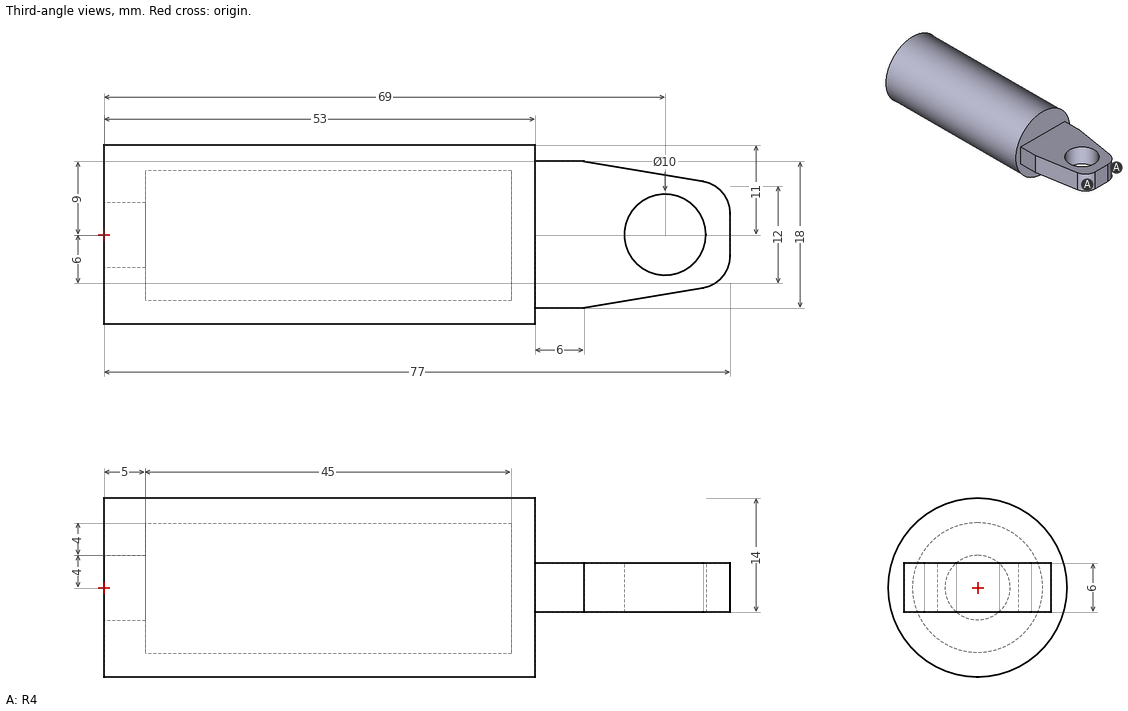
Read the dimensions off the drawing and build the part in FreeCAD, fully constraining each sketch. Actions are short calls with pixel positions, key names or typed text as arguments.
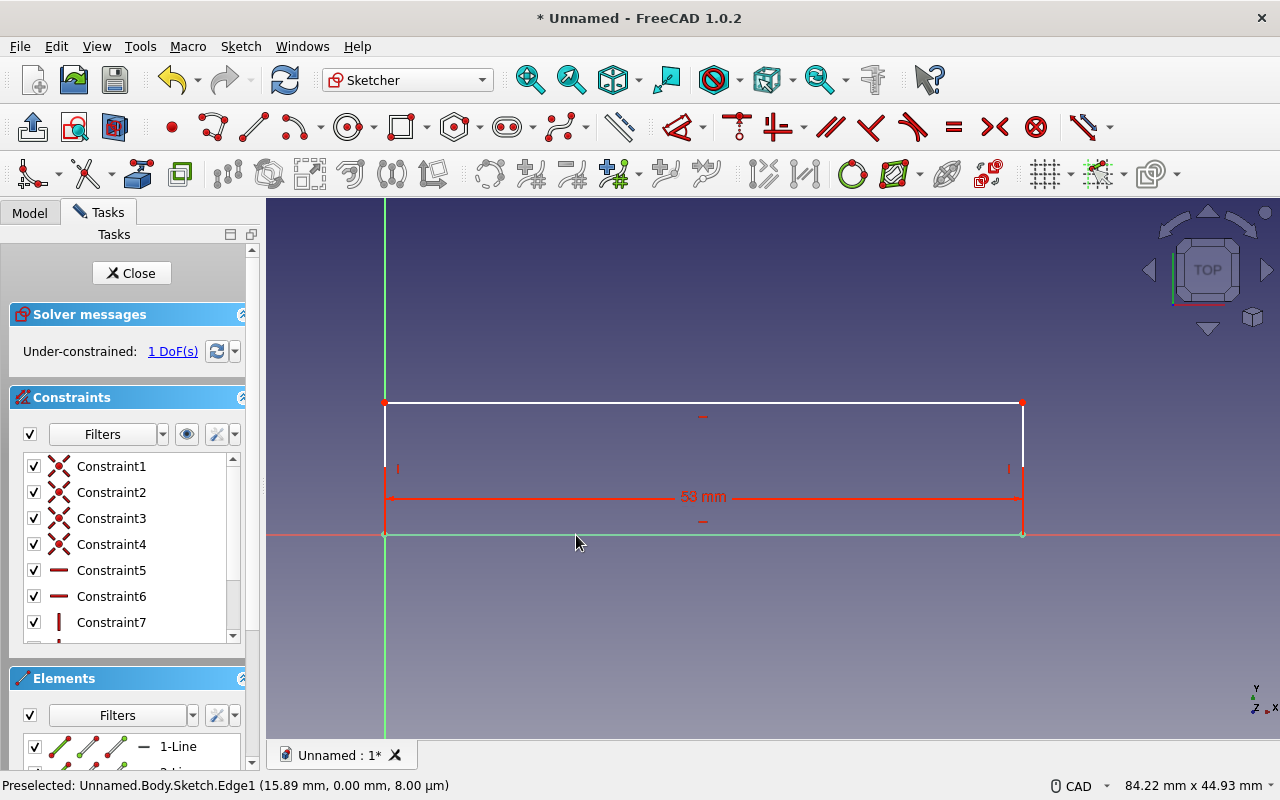
click(1023, 495)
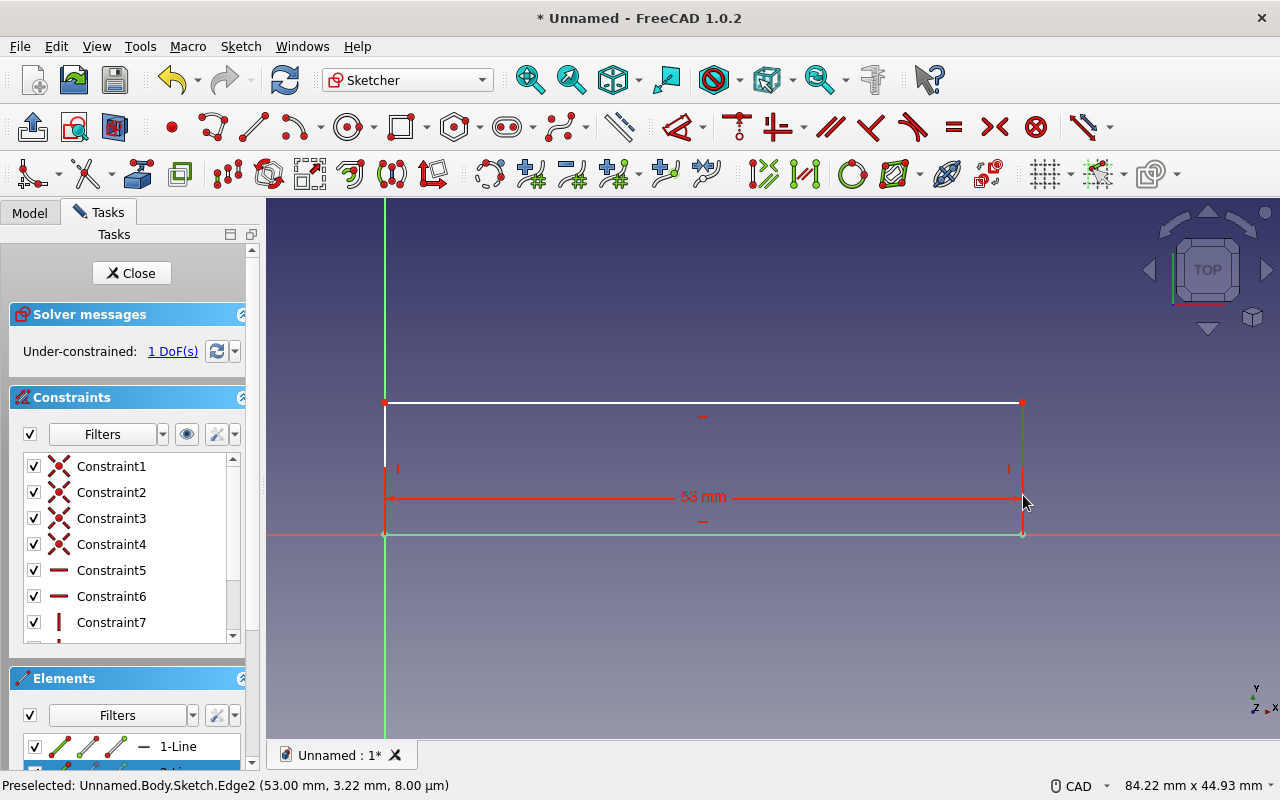
key(i)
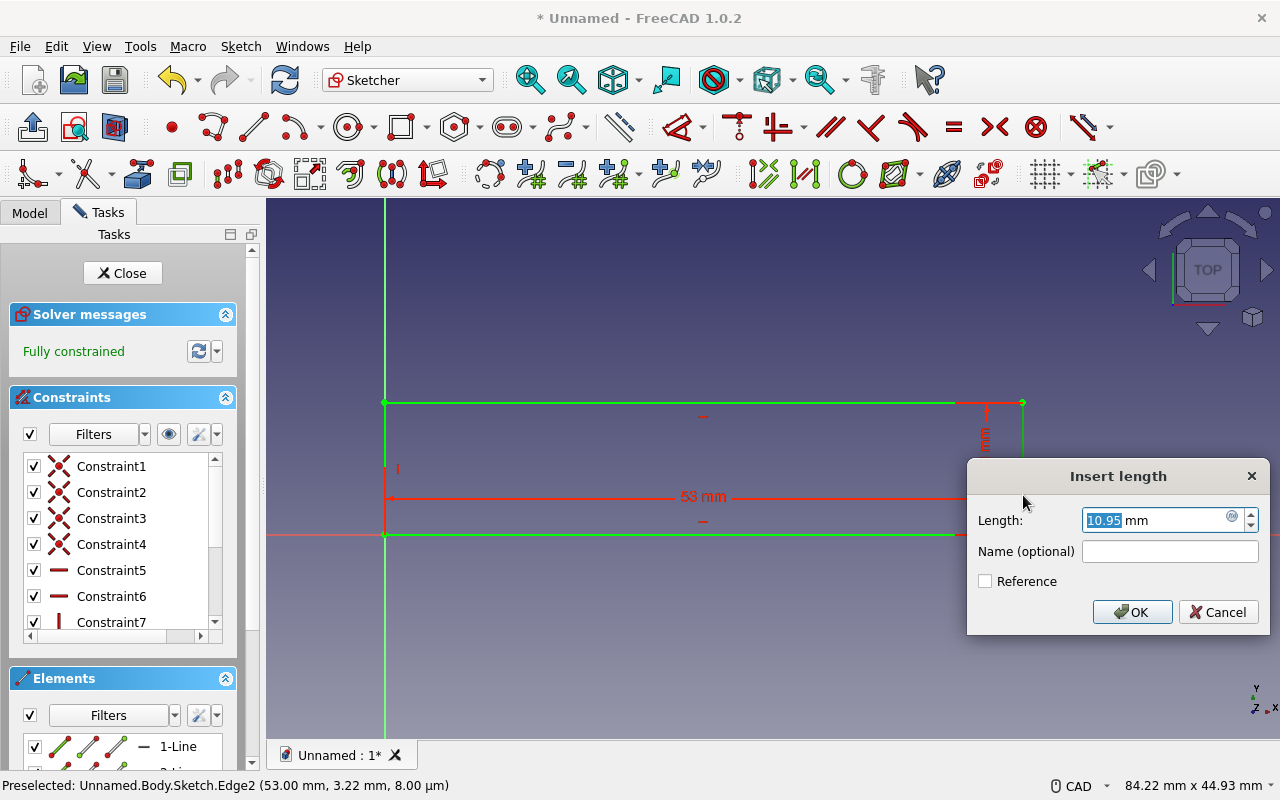
text(11)
key(Return)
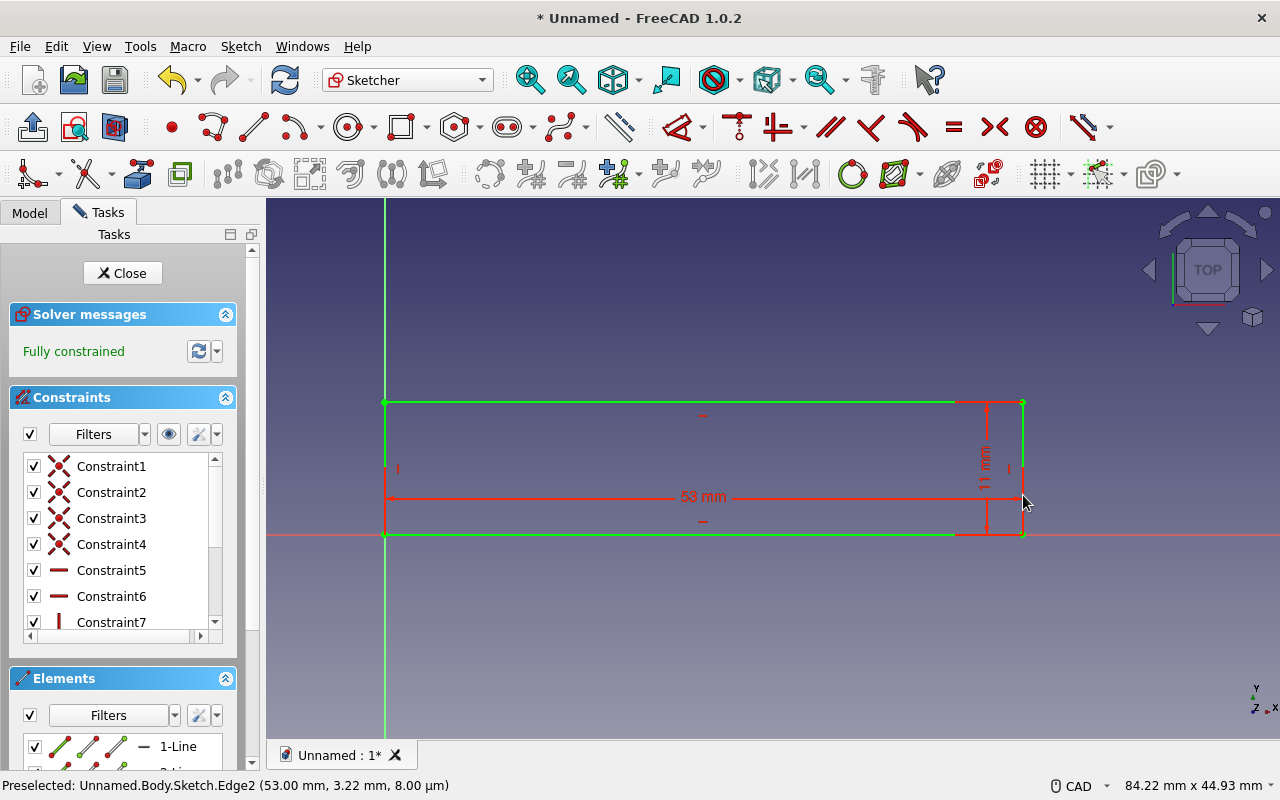
click(123, 273)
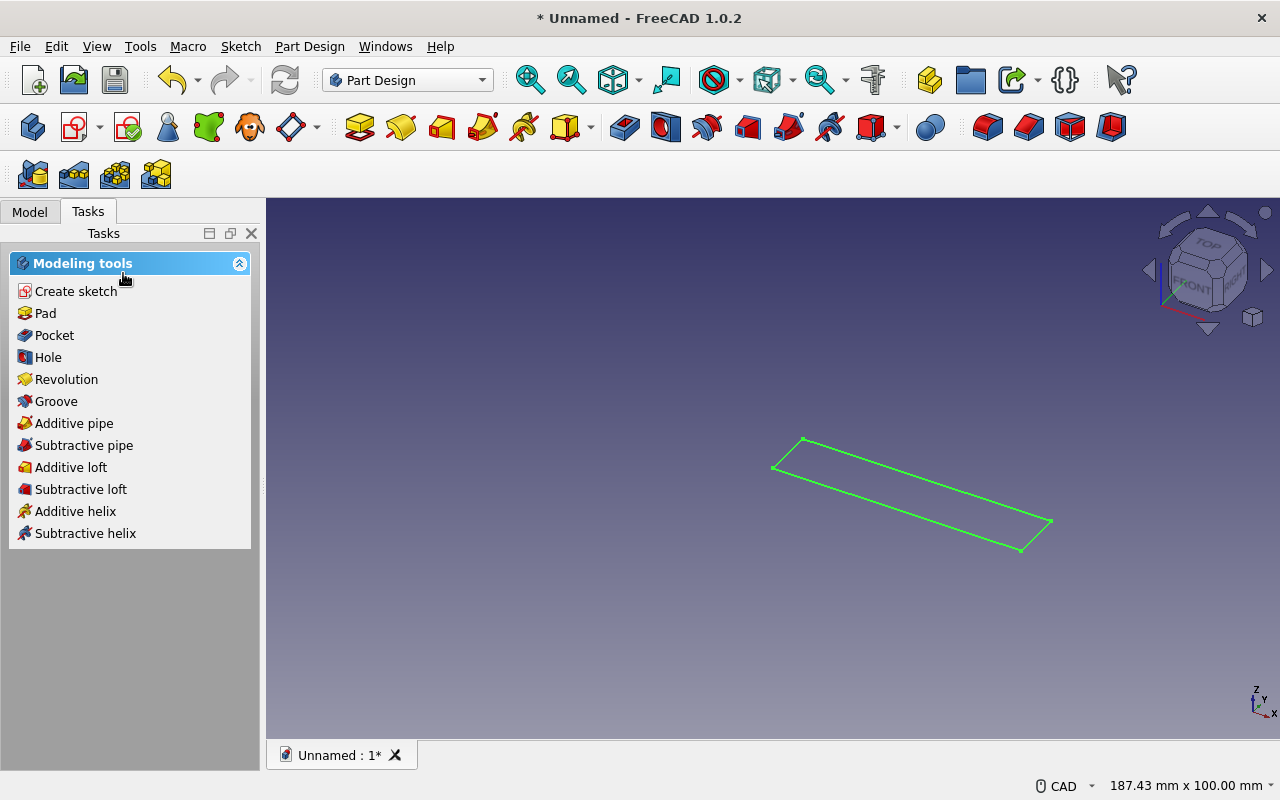
click(401, 128)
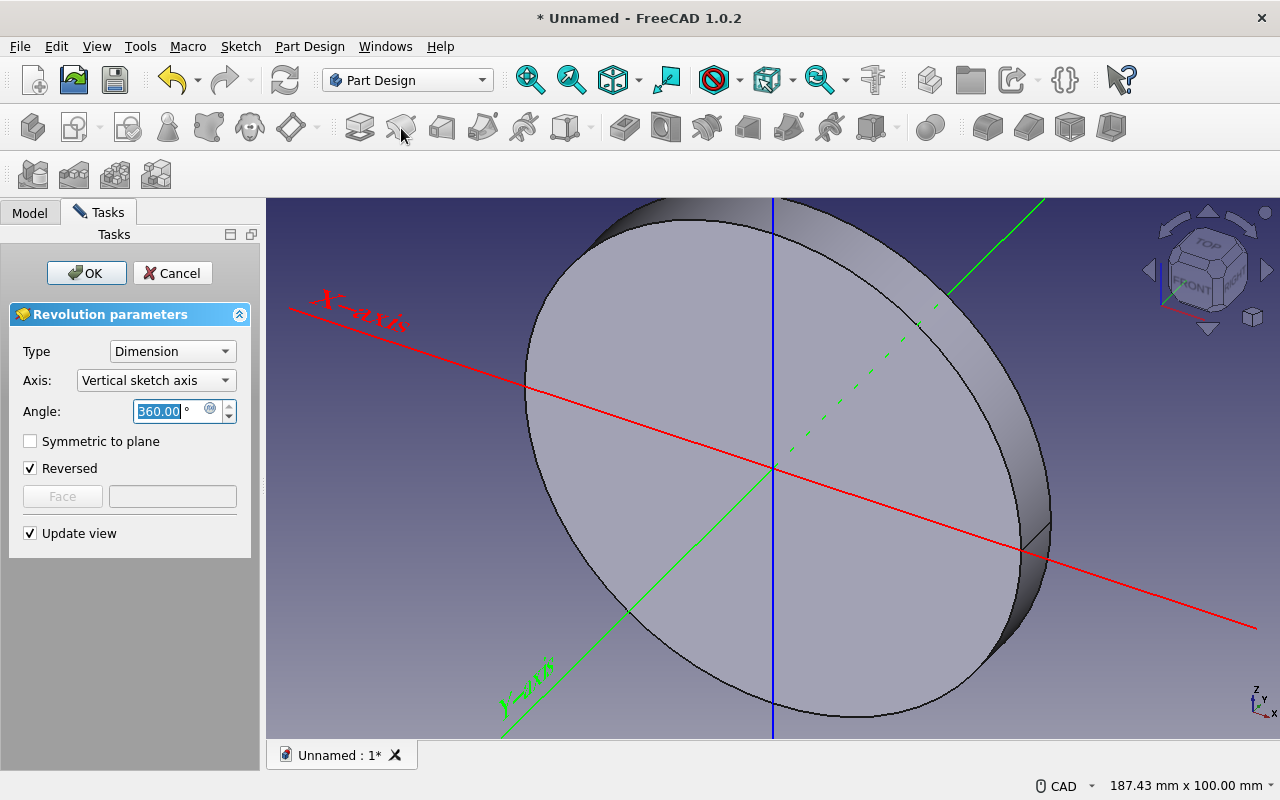
click(157, 380)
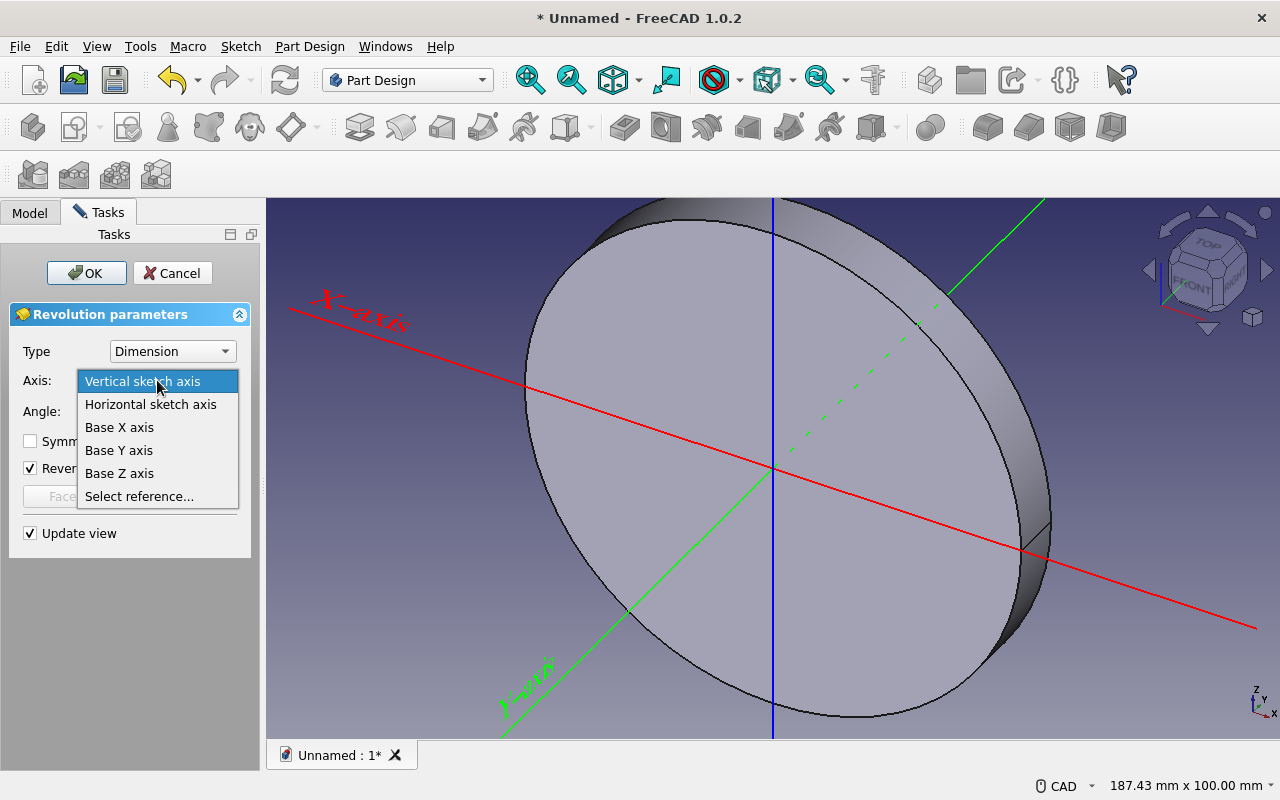
click(156, 404)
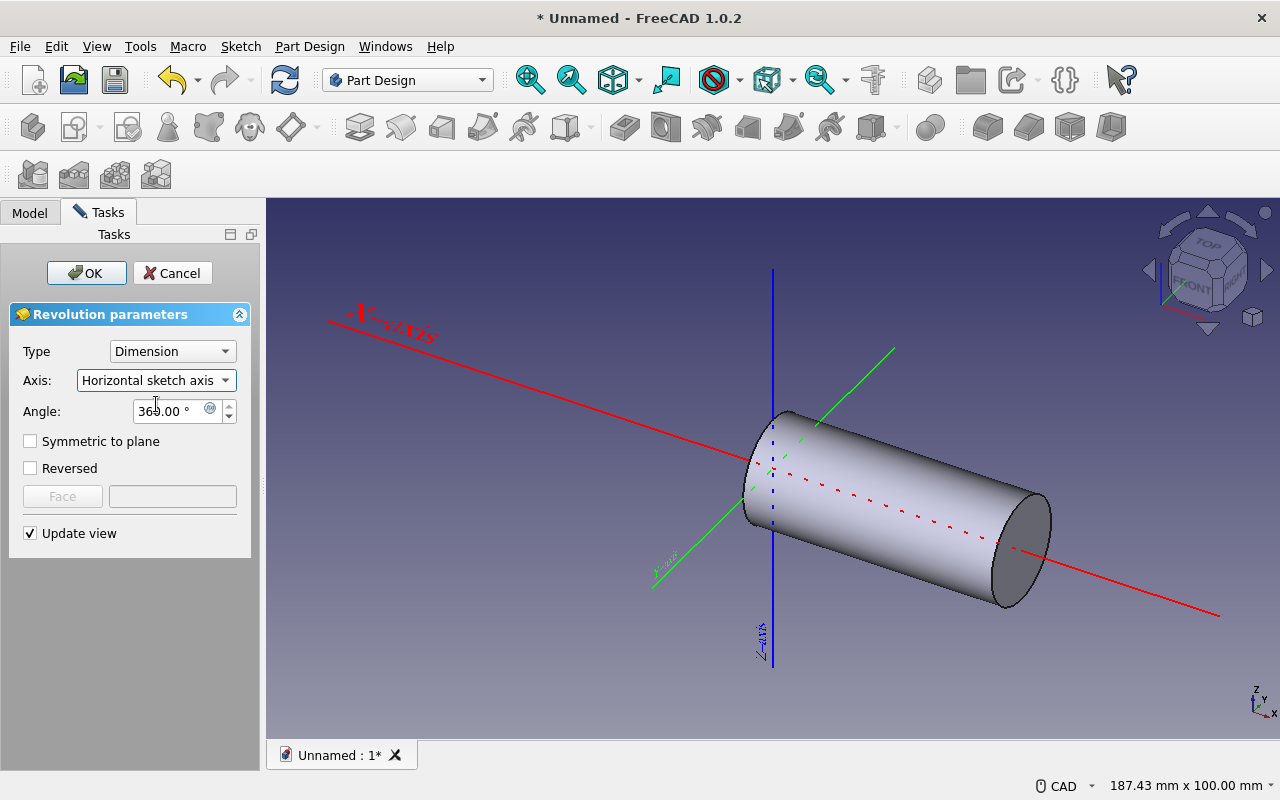
click(87, 273)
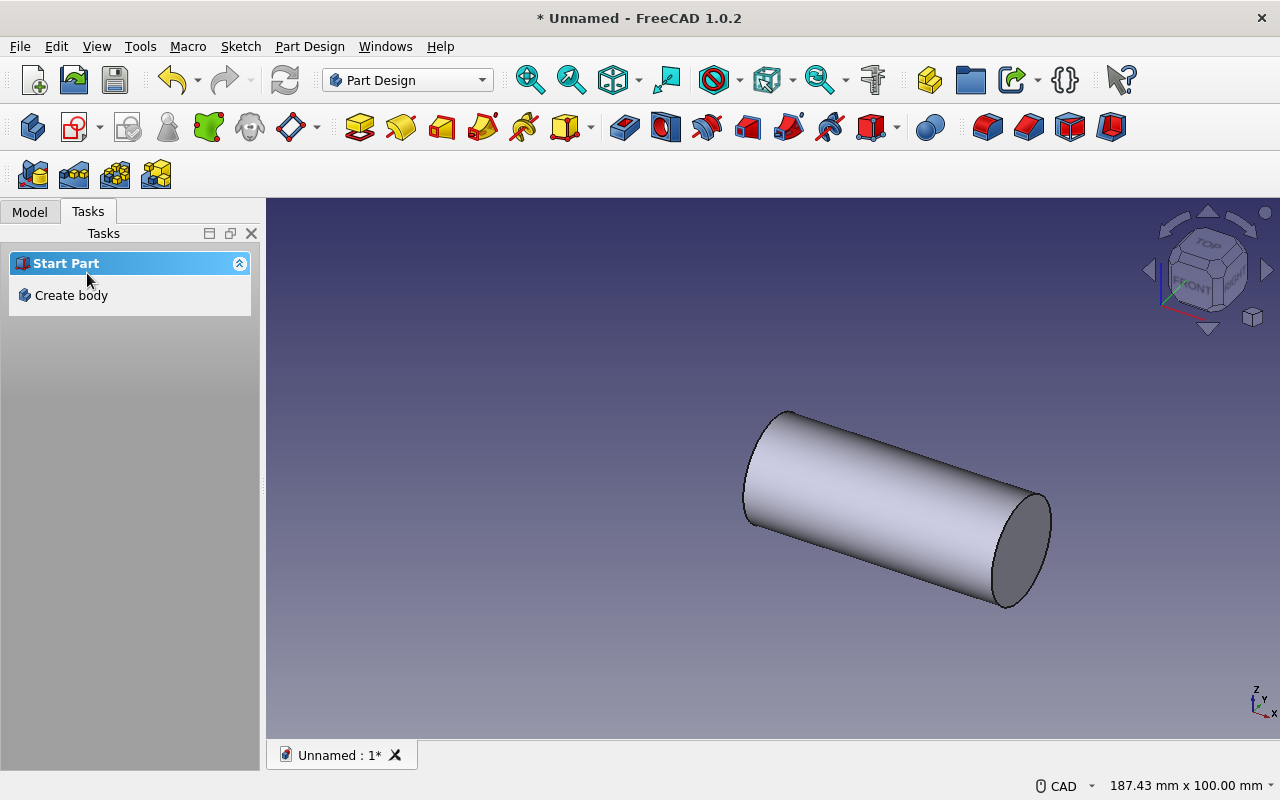
click(531, 80)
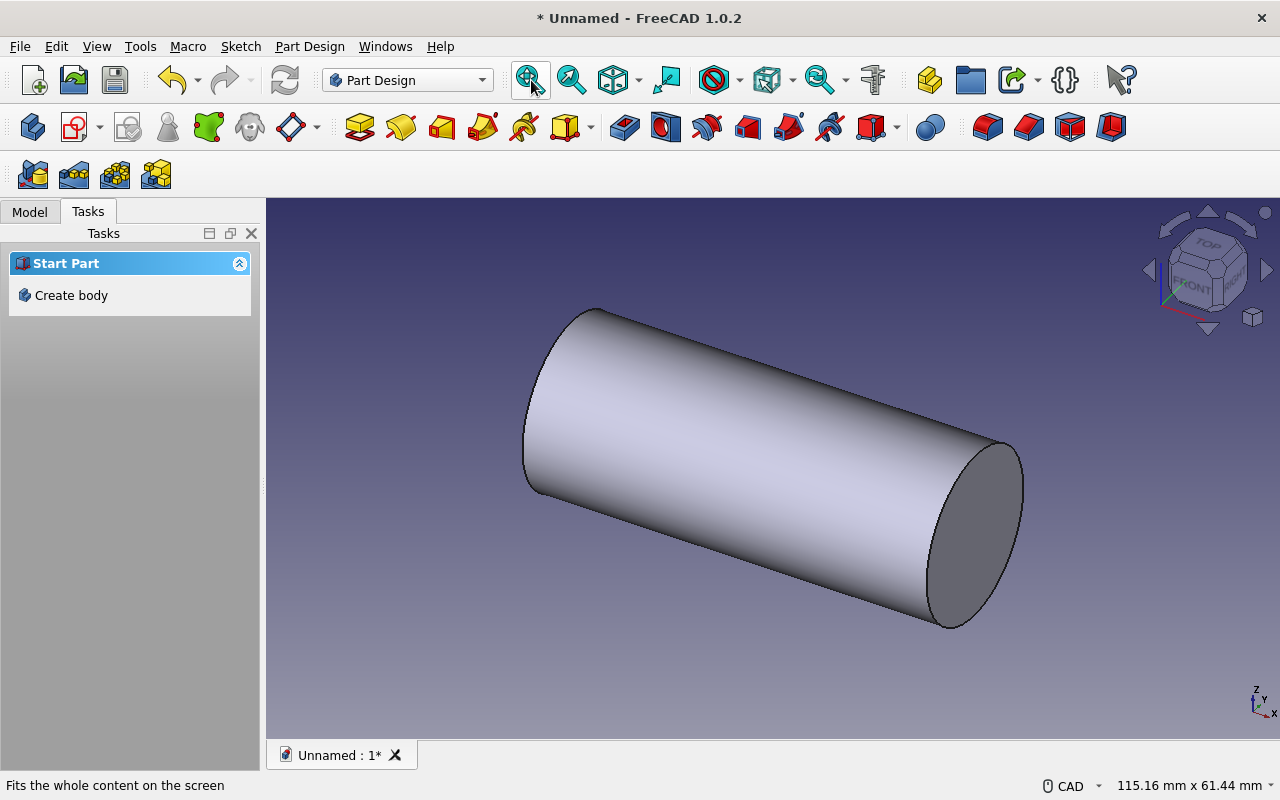
click(30, 212)